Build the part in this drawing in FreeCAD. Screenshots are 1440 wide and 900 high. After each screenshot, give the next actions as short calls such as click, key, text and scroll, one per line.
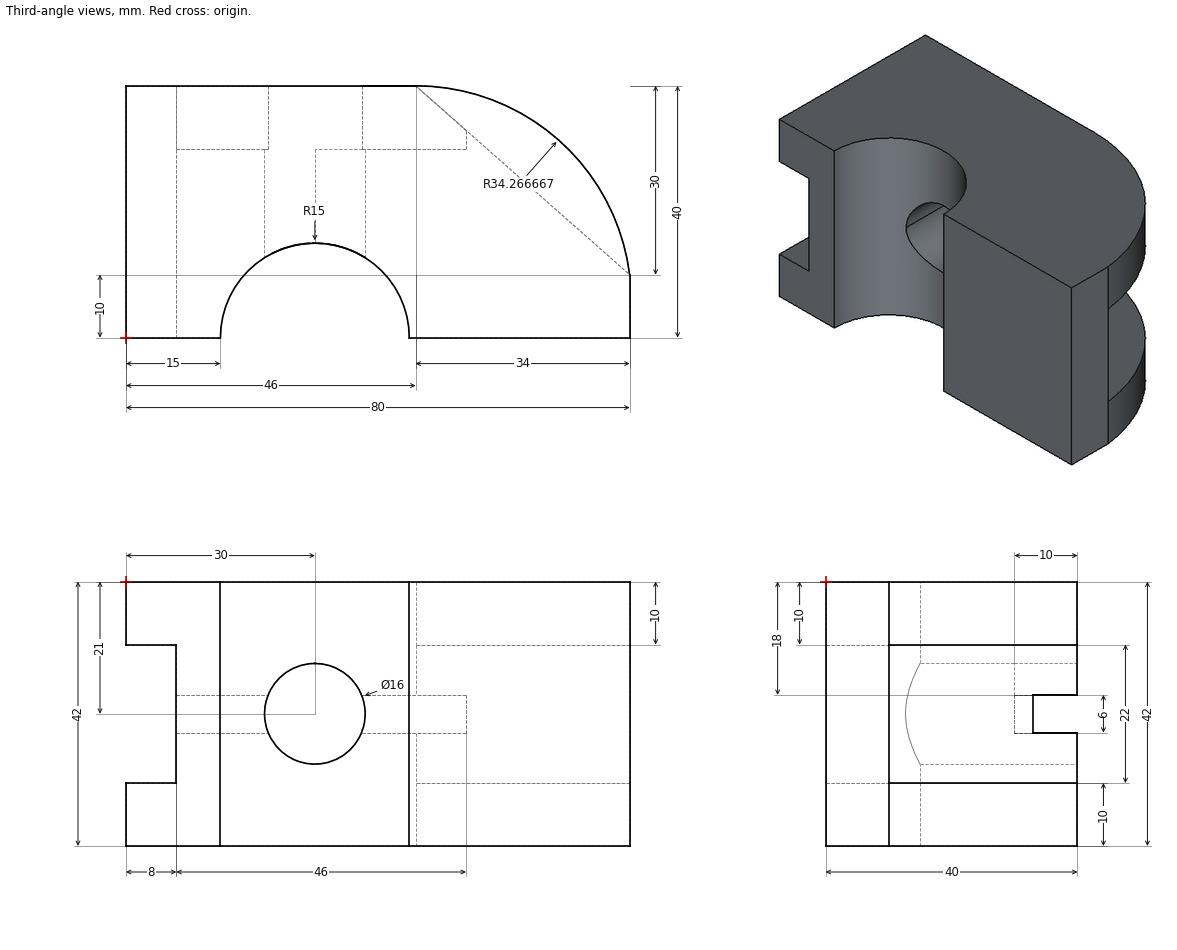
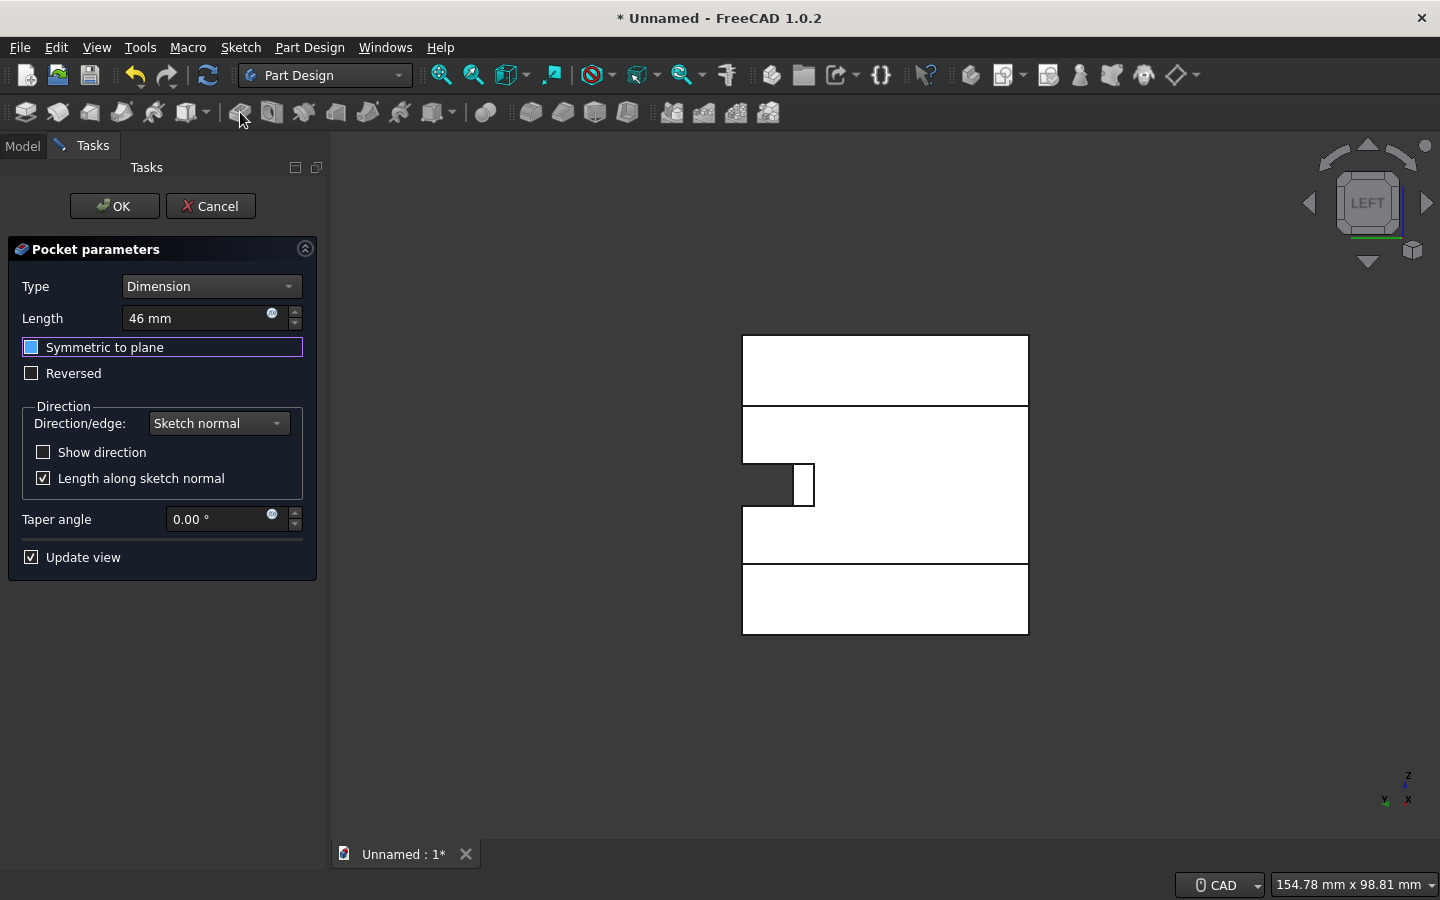
click(115, 206)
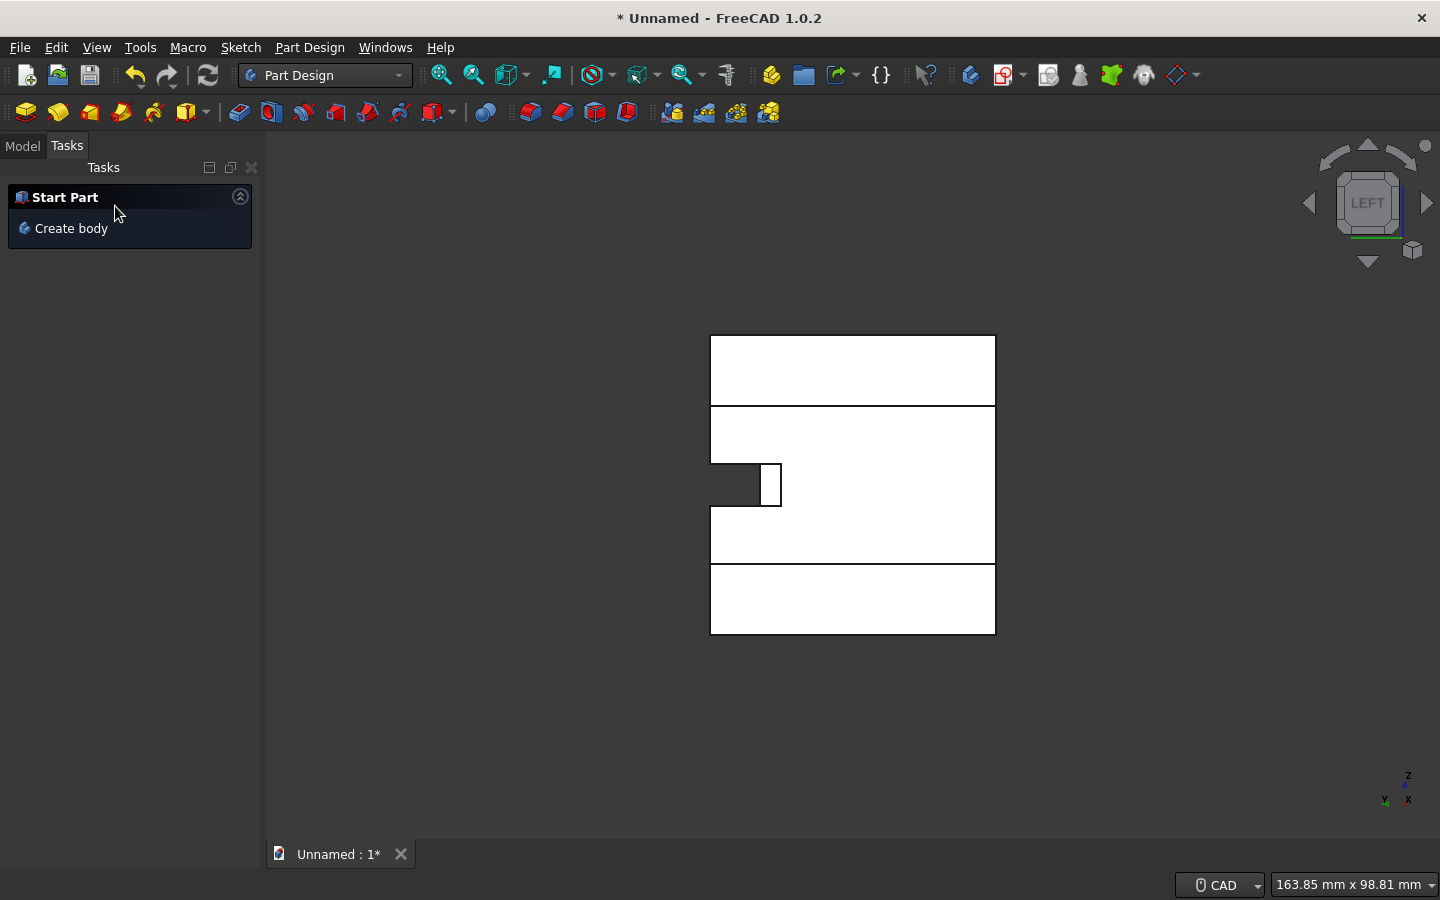
click(442, 76)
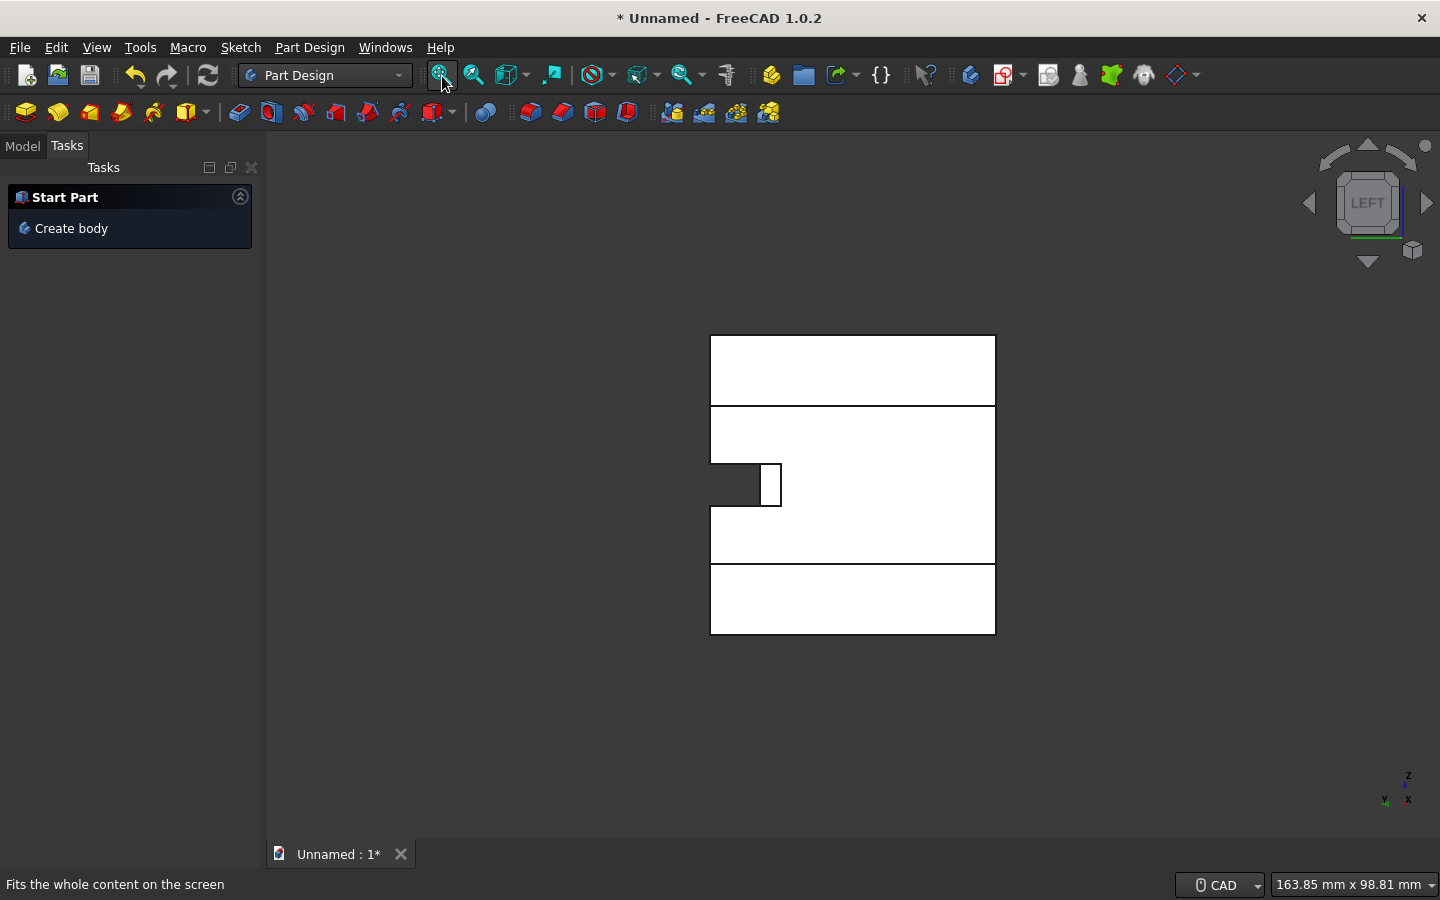
key(4)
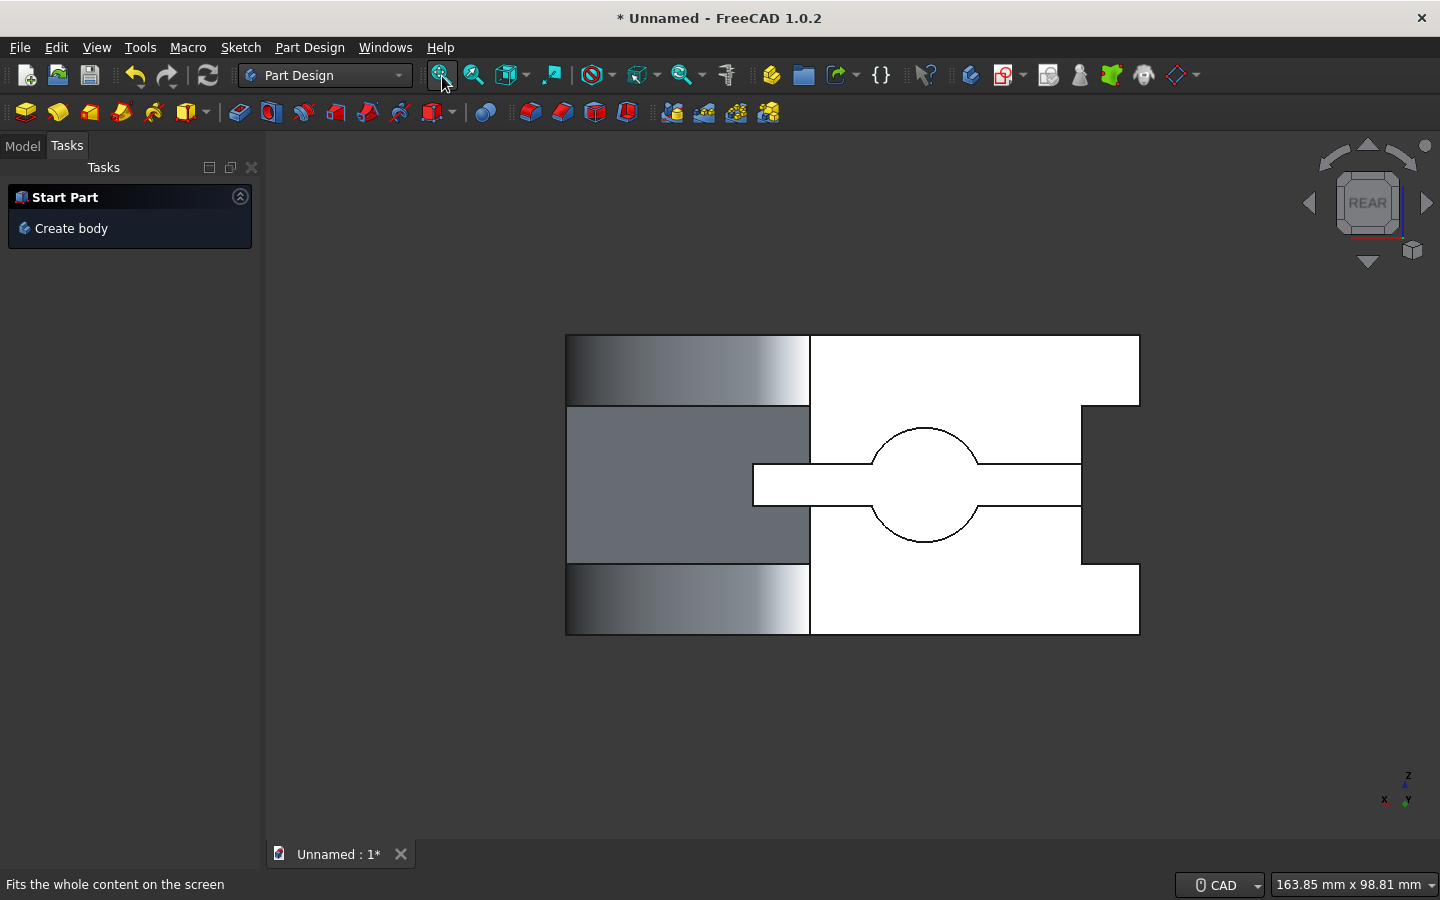
click(917, 484)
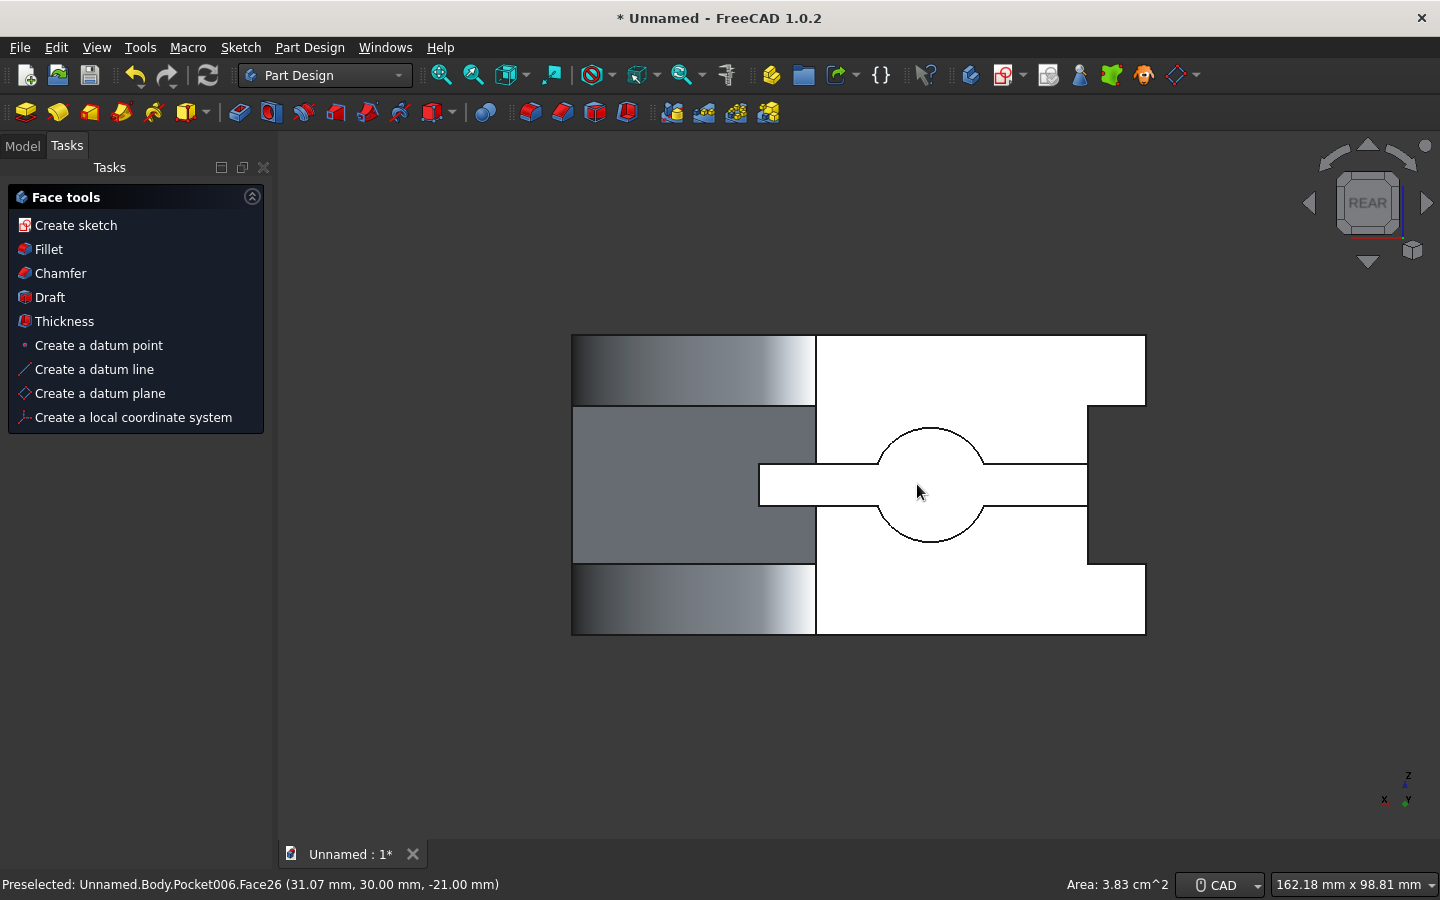
click(1004, 76)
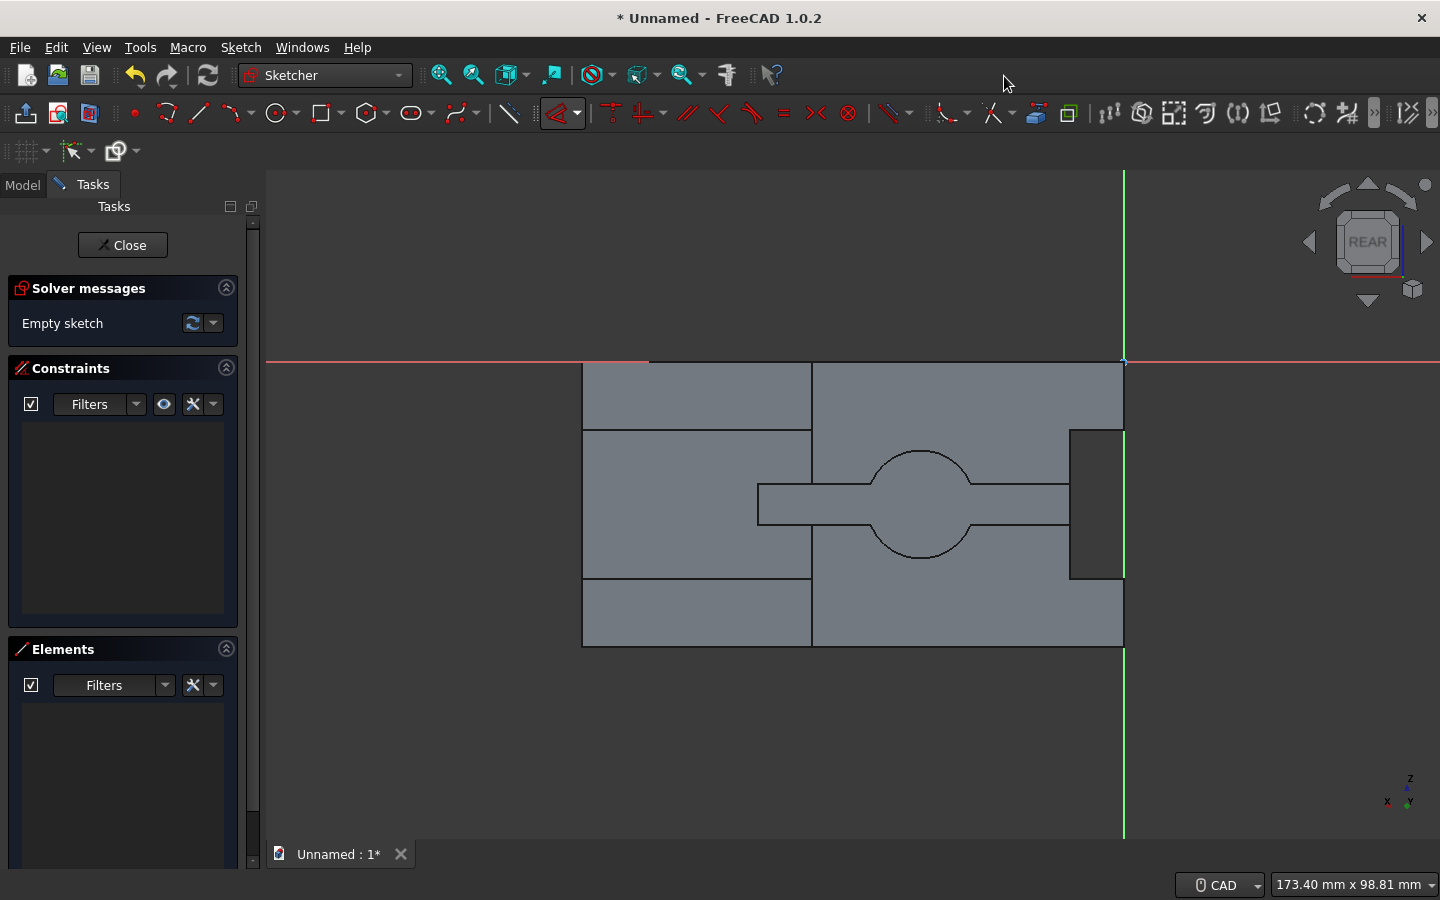
click(90, 114)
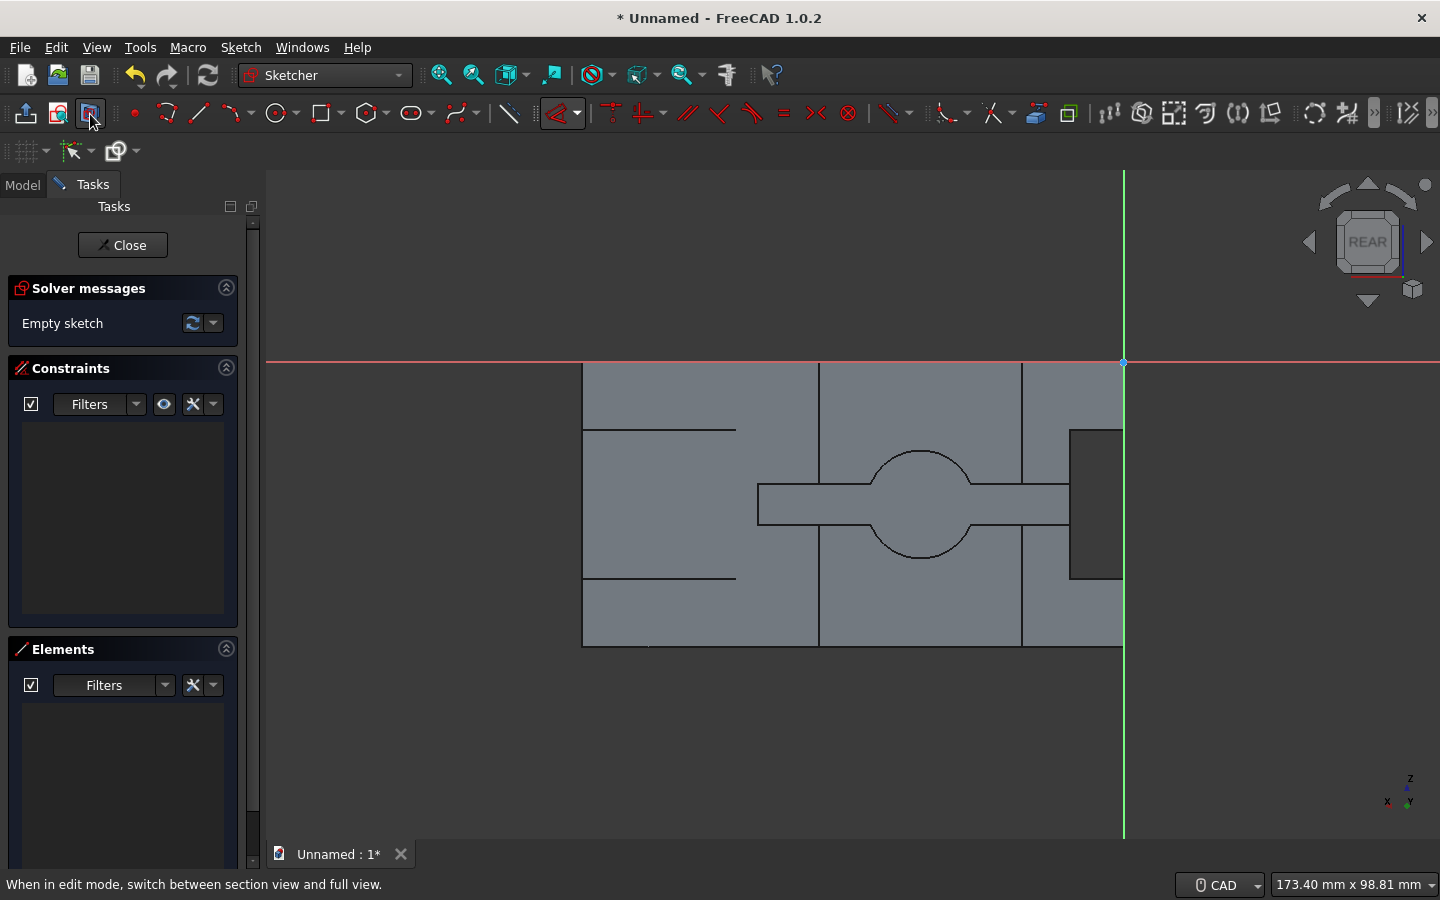
scroll(1167, 425, up, 4)